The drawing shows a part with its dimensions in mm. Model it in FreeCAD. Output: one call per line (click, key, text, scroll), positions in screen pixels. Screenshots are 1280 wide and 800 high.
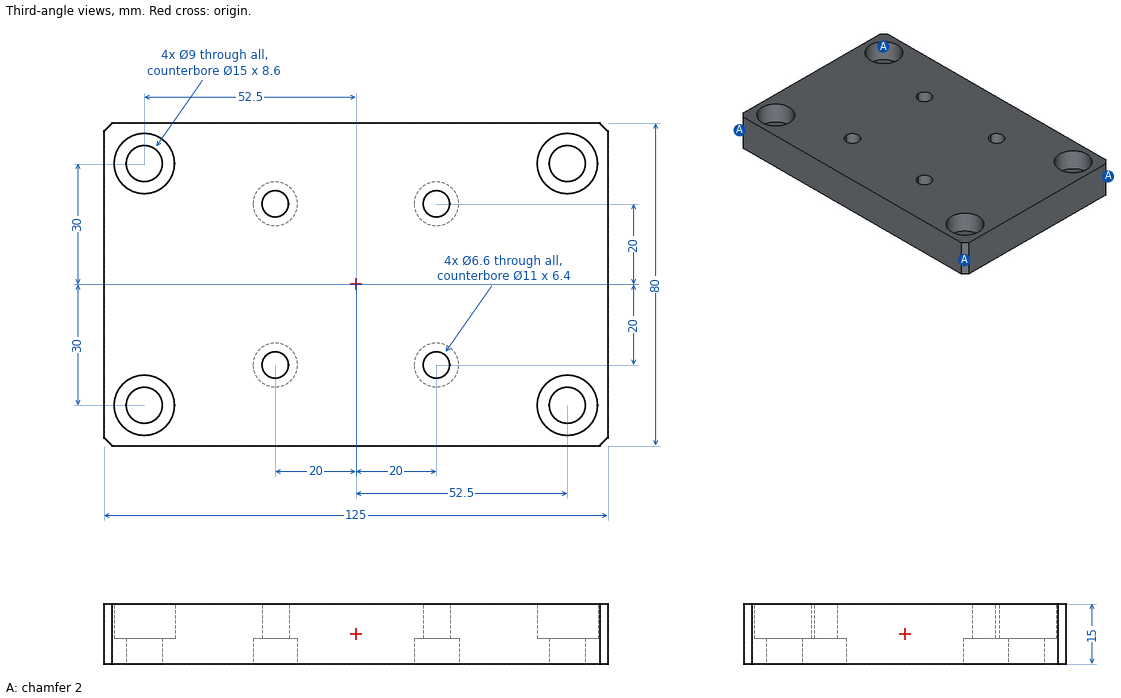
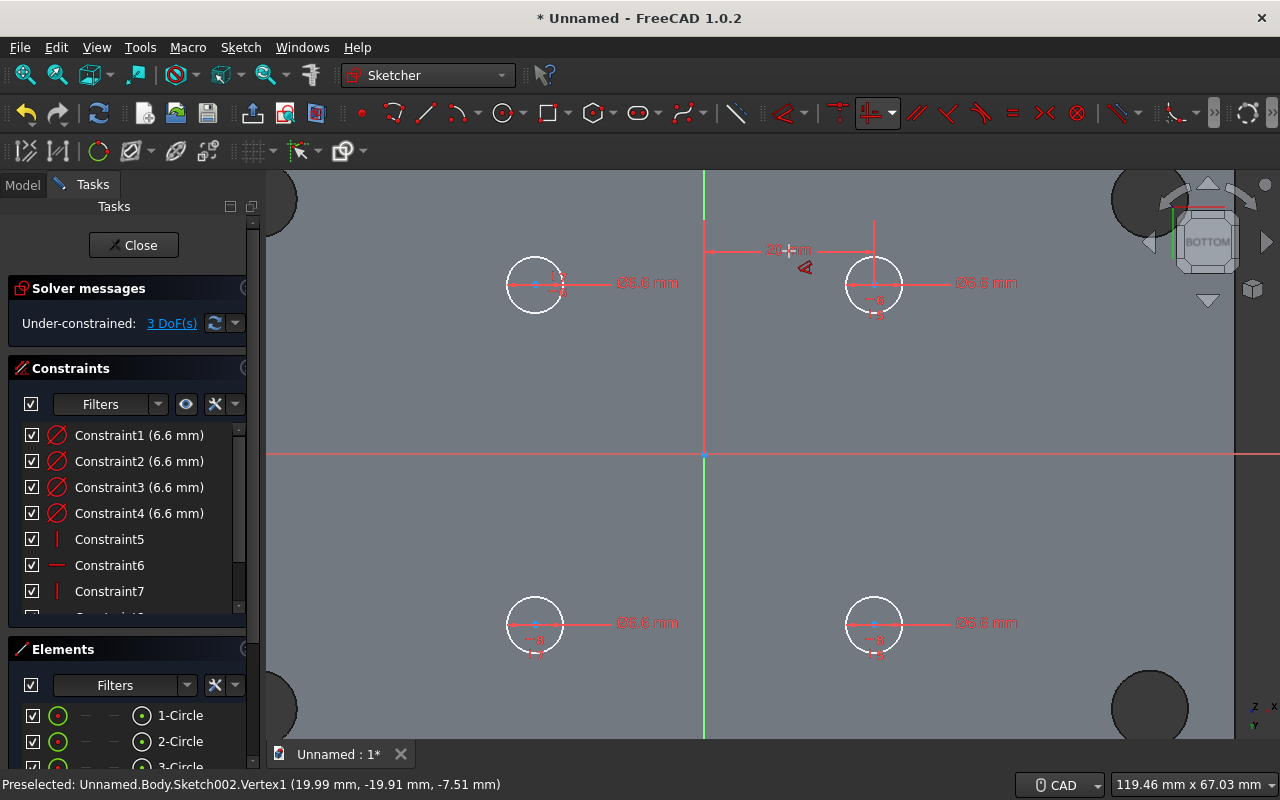
click(874, 285)
click(908, 370)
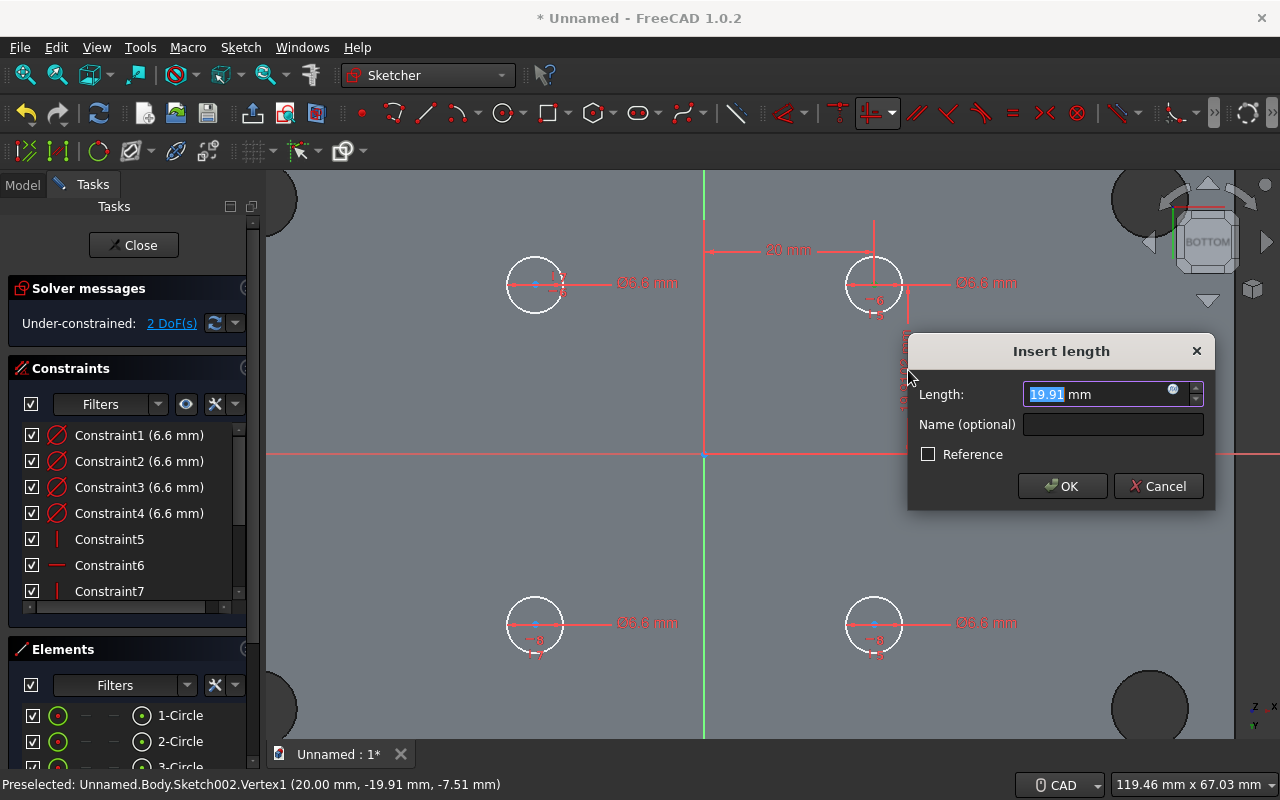
text(20)
key(Return)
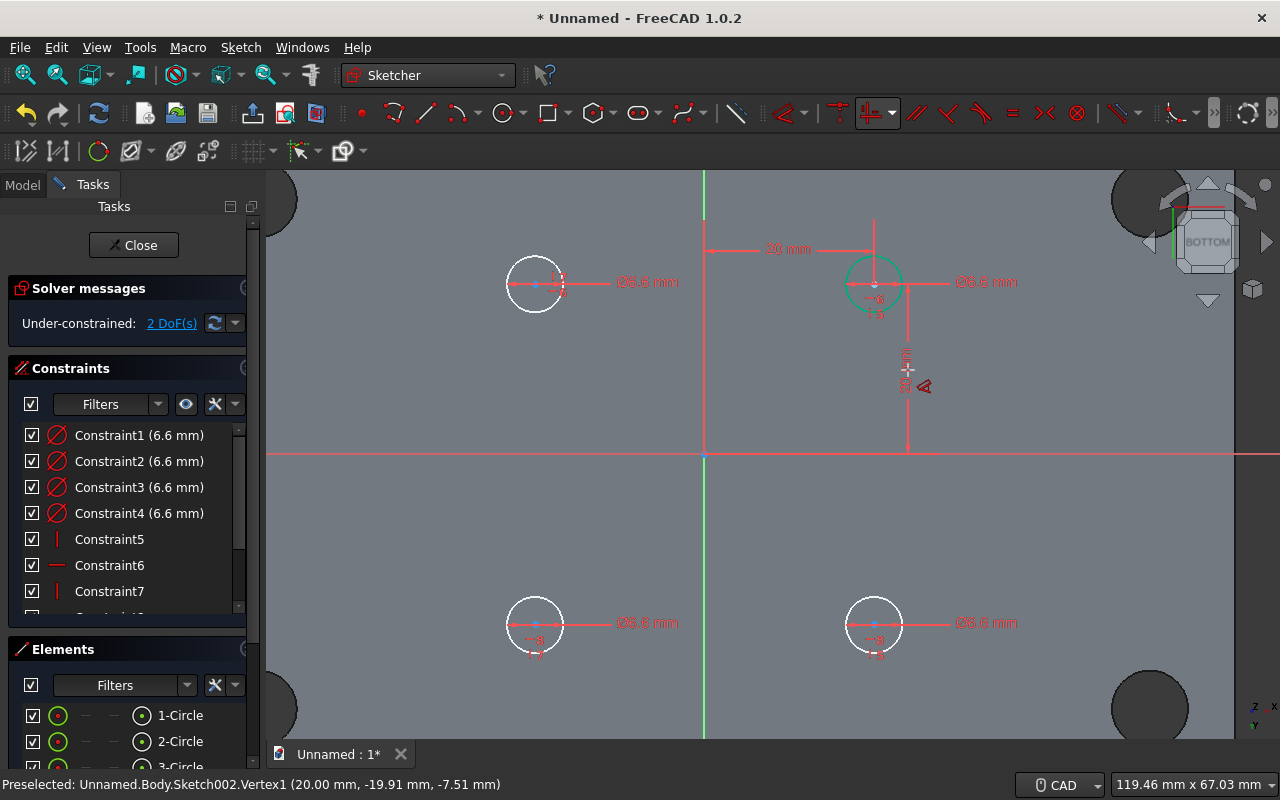
click(874, 625)
click(908, 540)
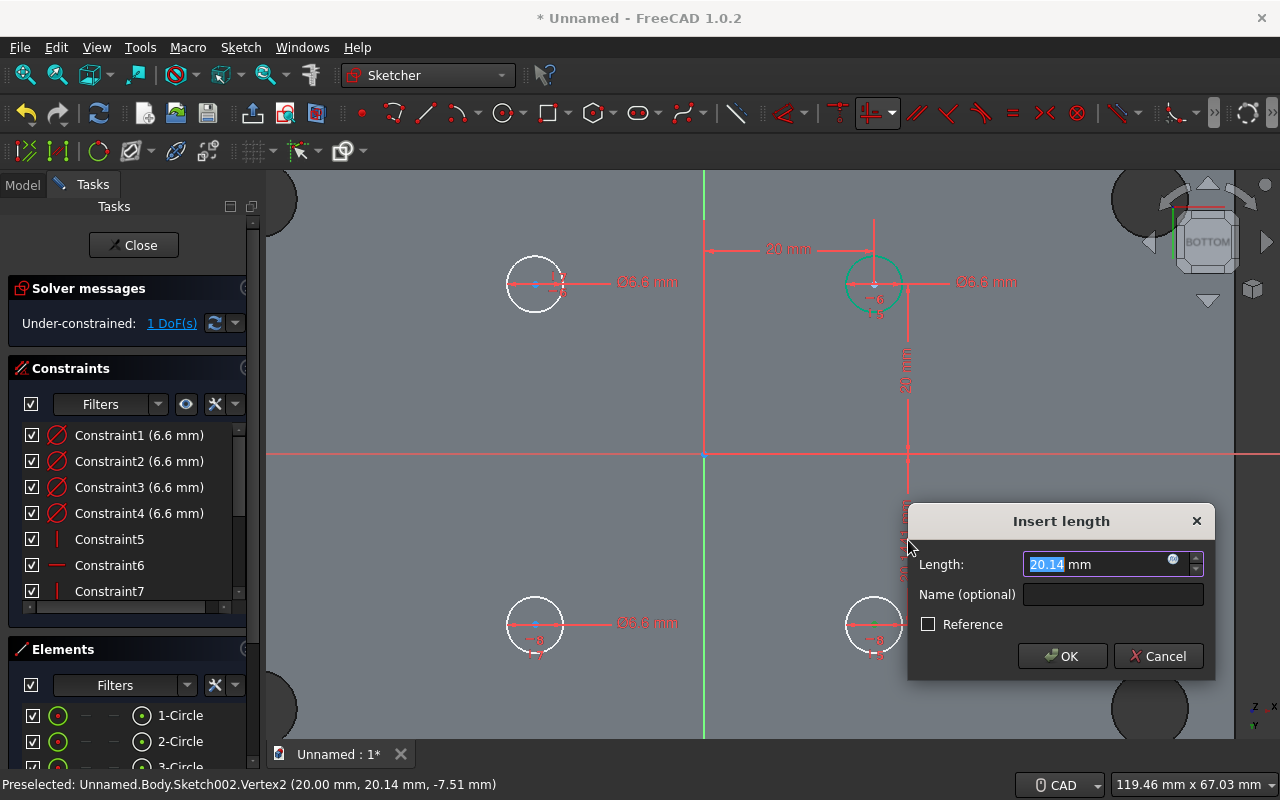
text(20)
key(Return)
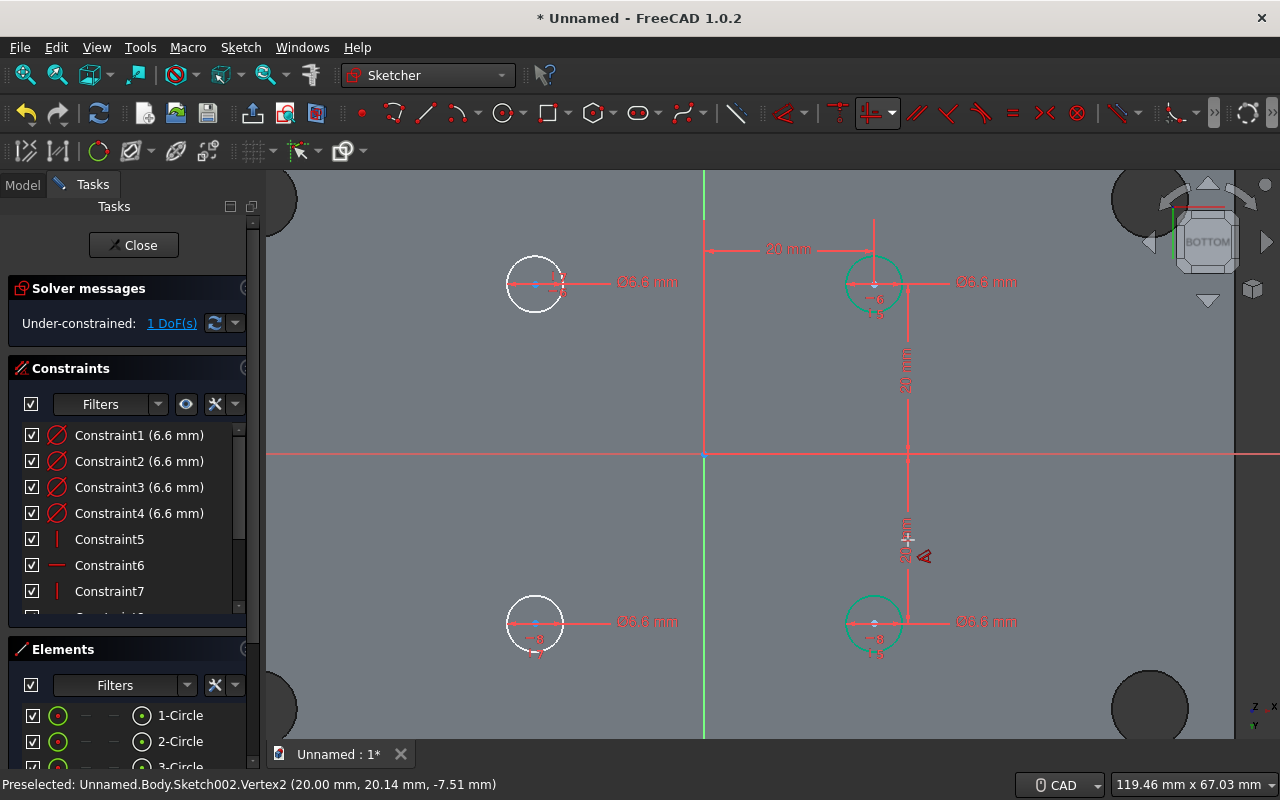
click(535, 284)
click(620, 250)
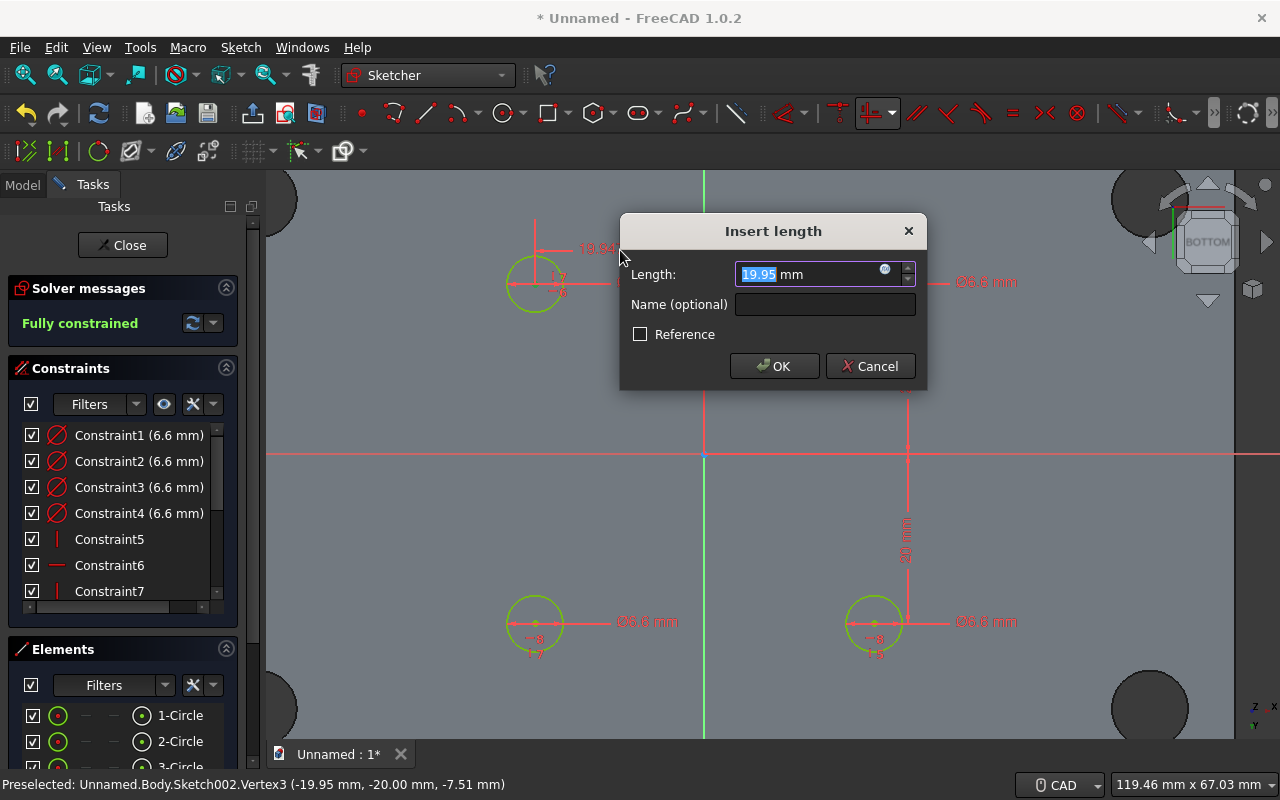
text(20)
key(Return)
key(Escape)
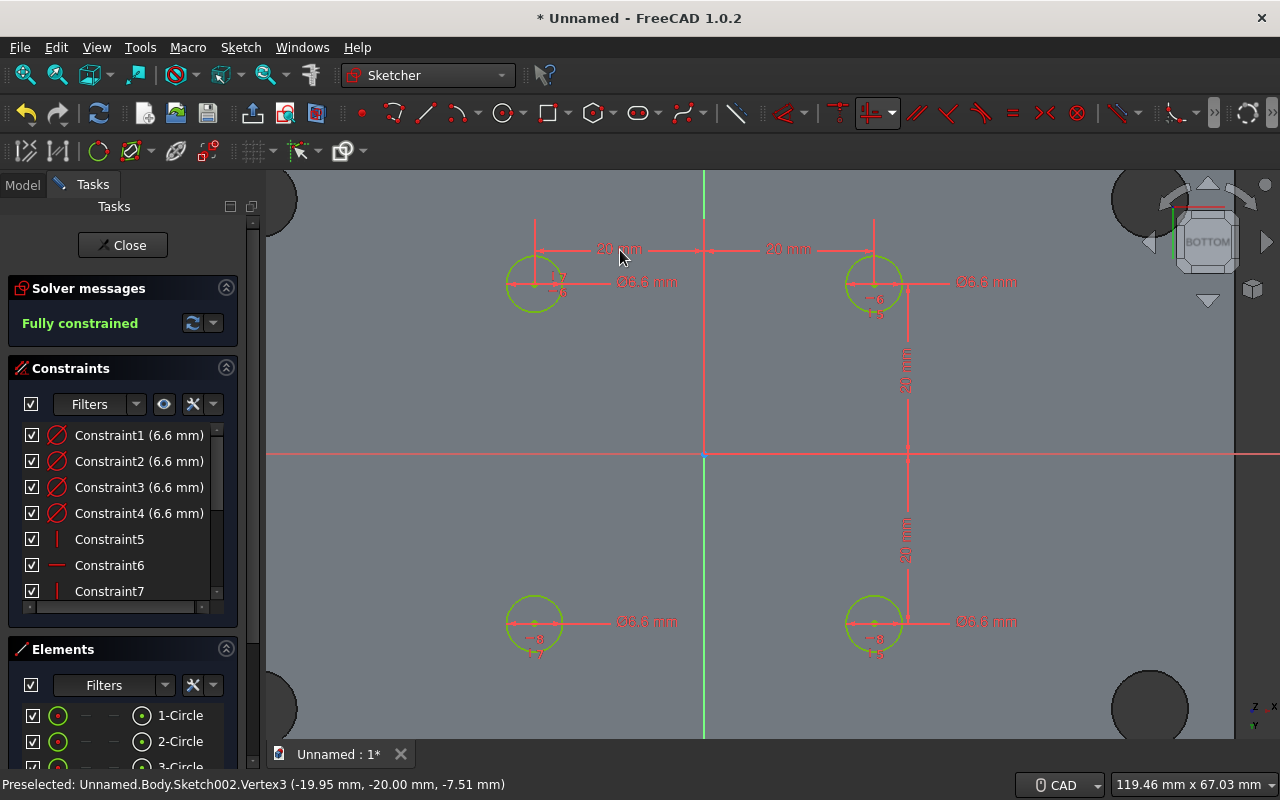
click(123, 245)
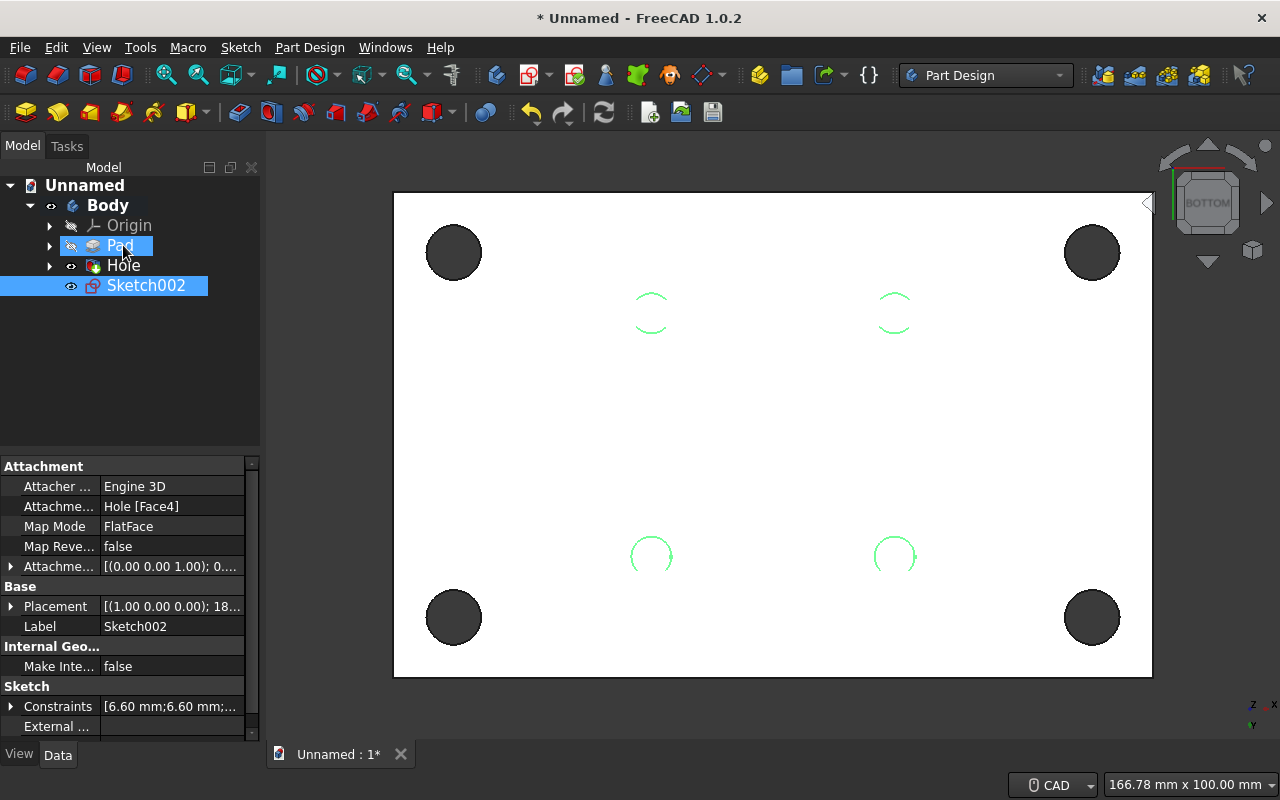
click(272, 112)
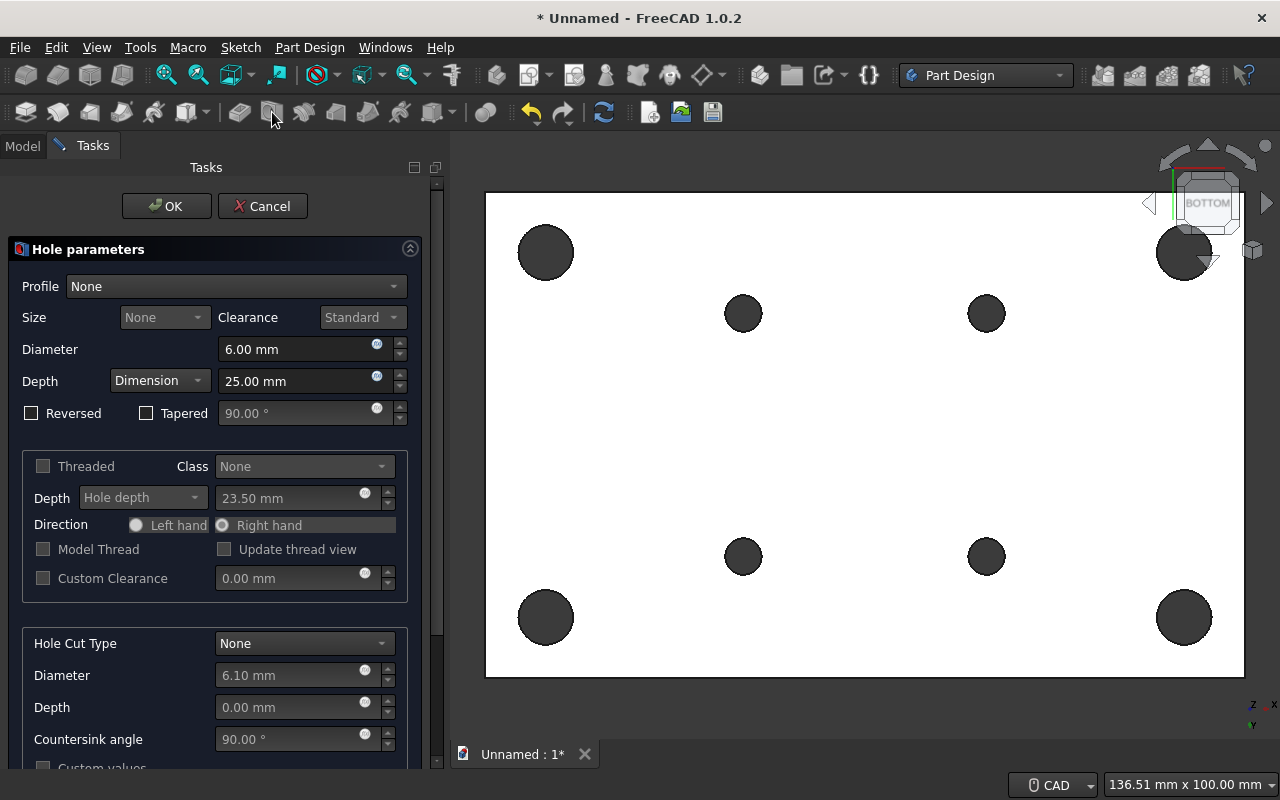
triple_click(305, 349)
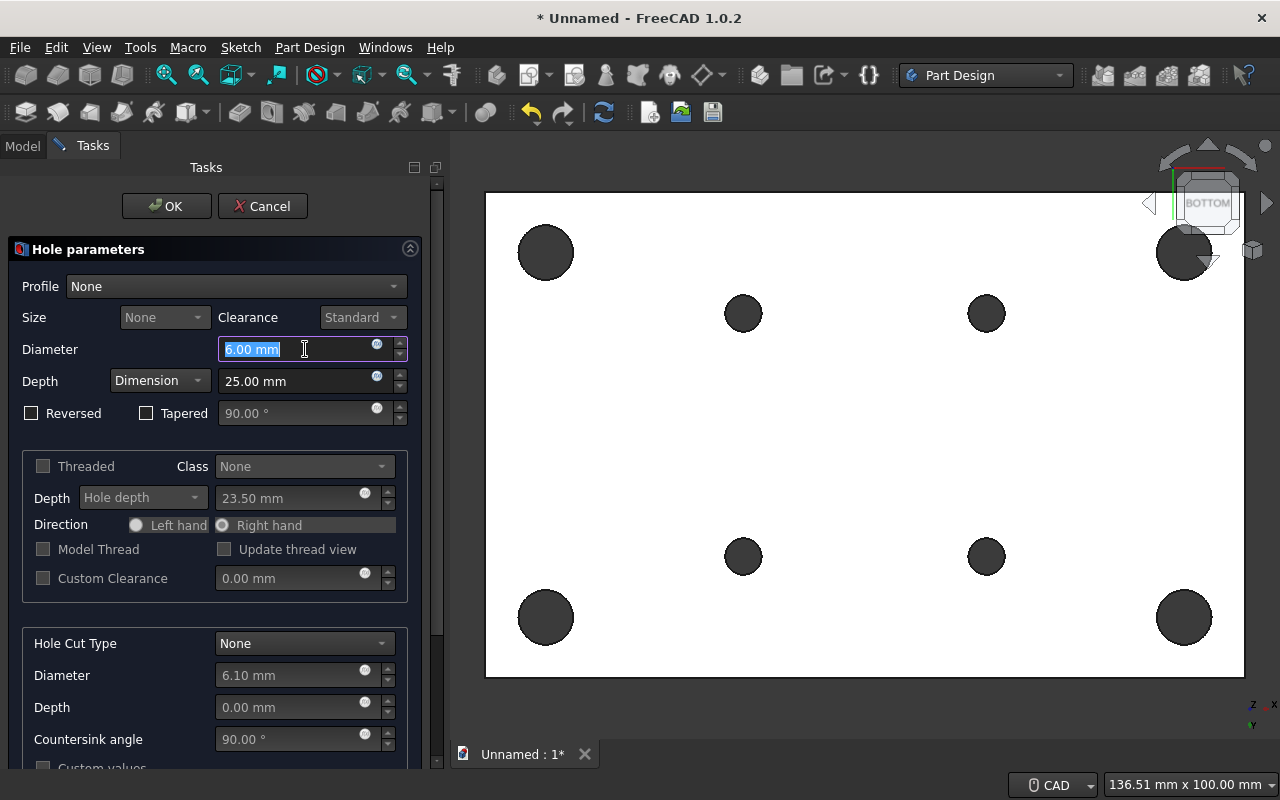
text(6.6)
key(Tab)